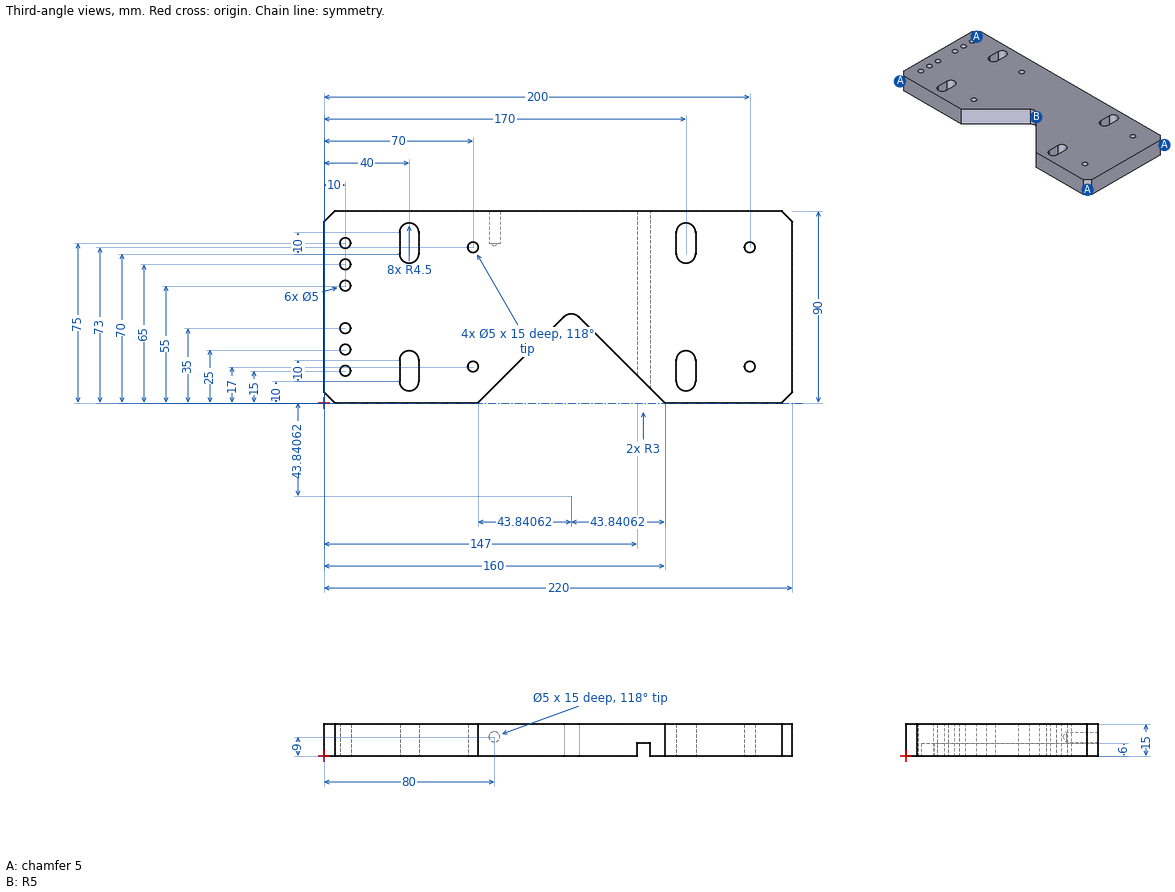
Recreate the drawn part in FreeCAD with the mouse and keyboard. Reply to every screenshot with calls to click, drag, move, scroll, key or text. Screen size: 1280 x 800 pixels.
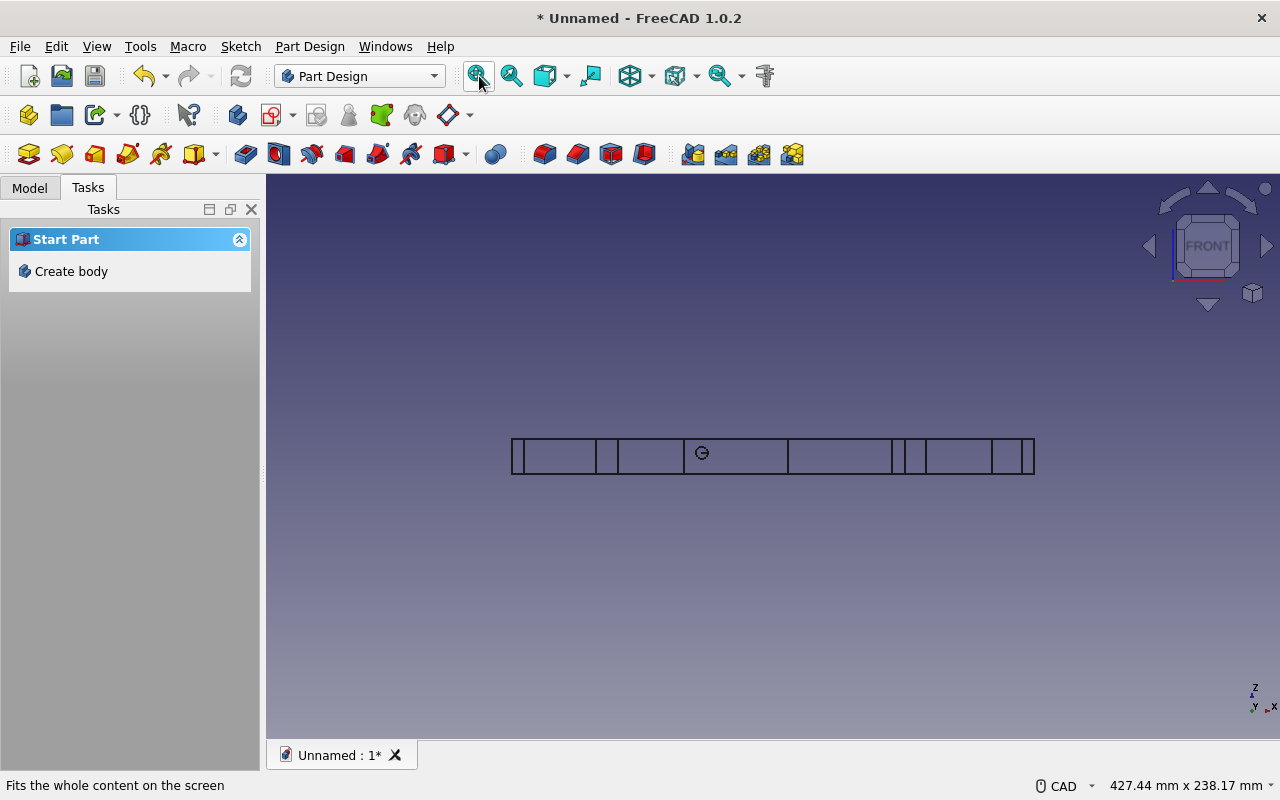
click(788, 455)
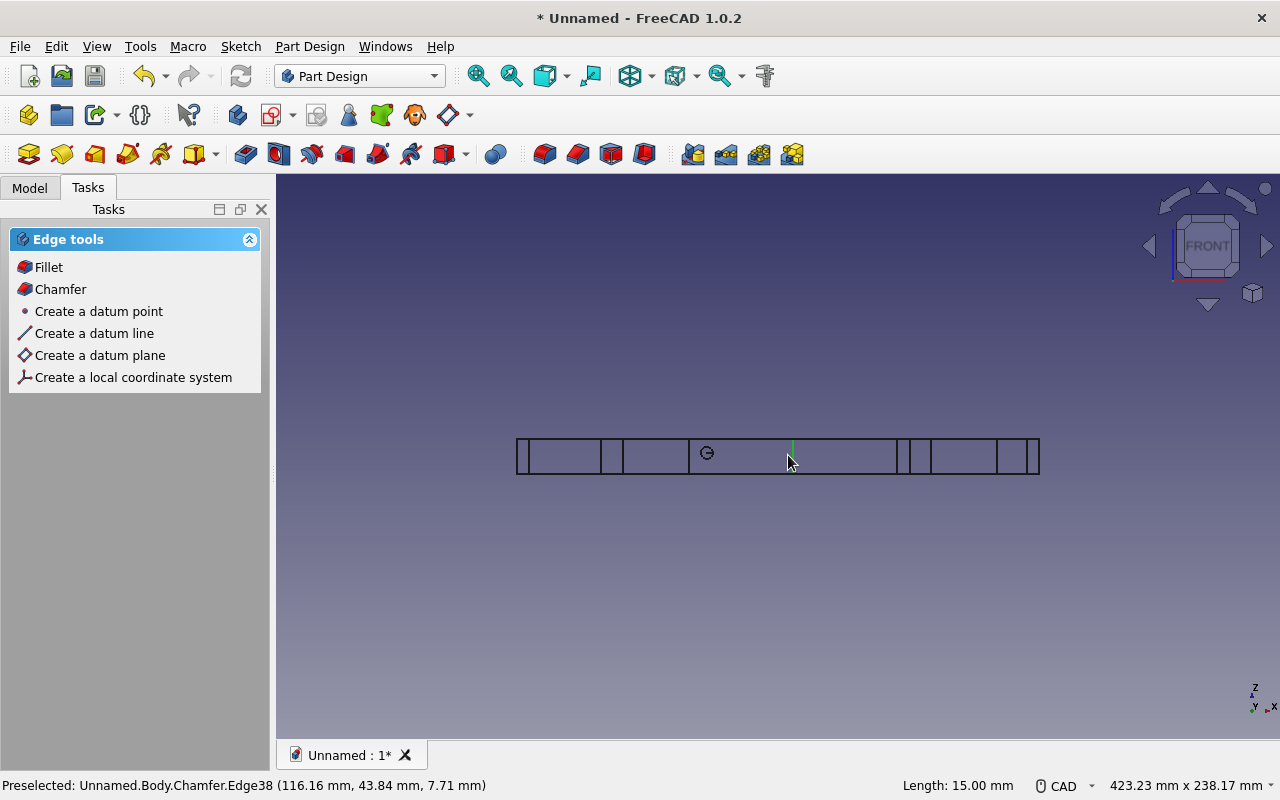
key(v)
key(1)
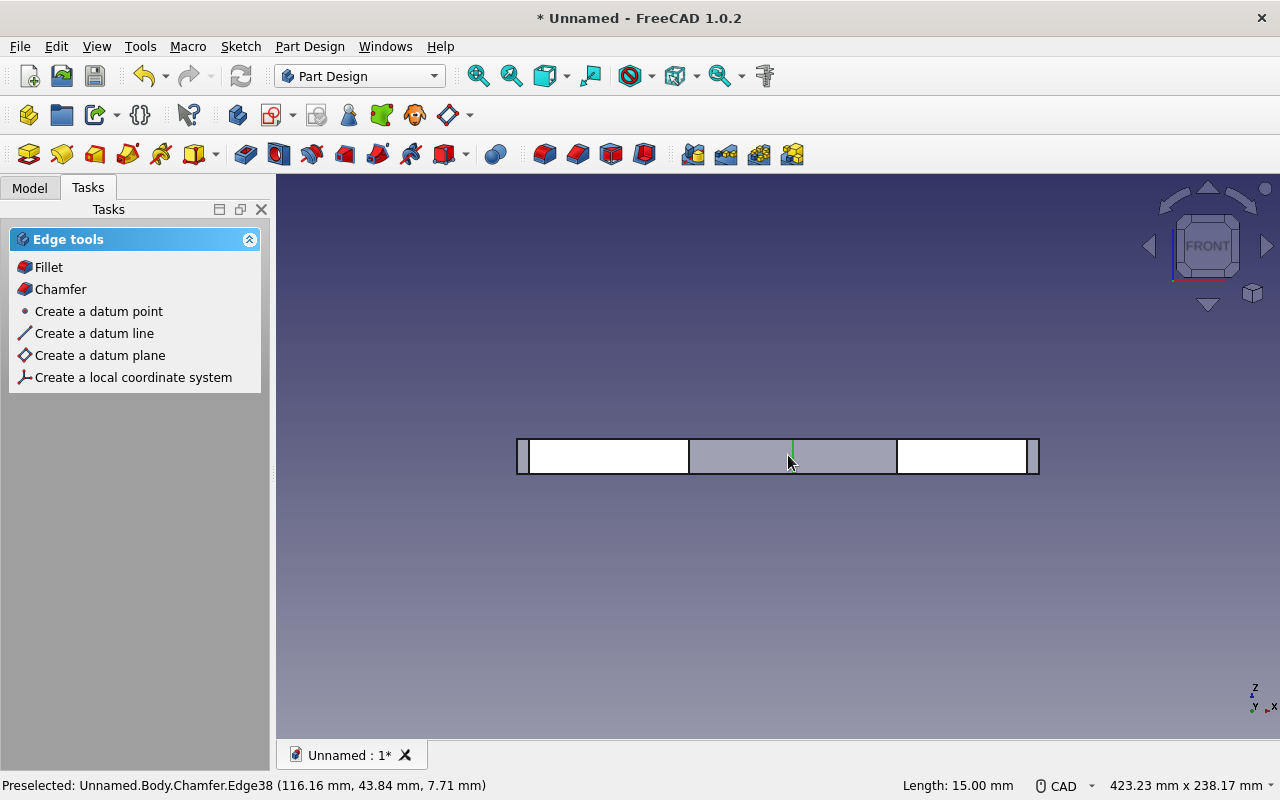
click(545, 154)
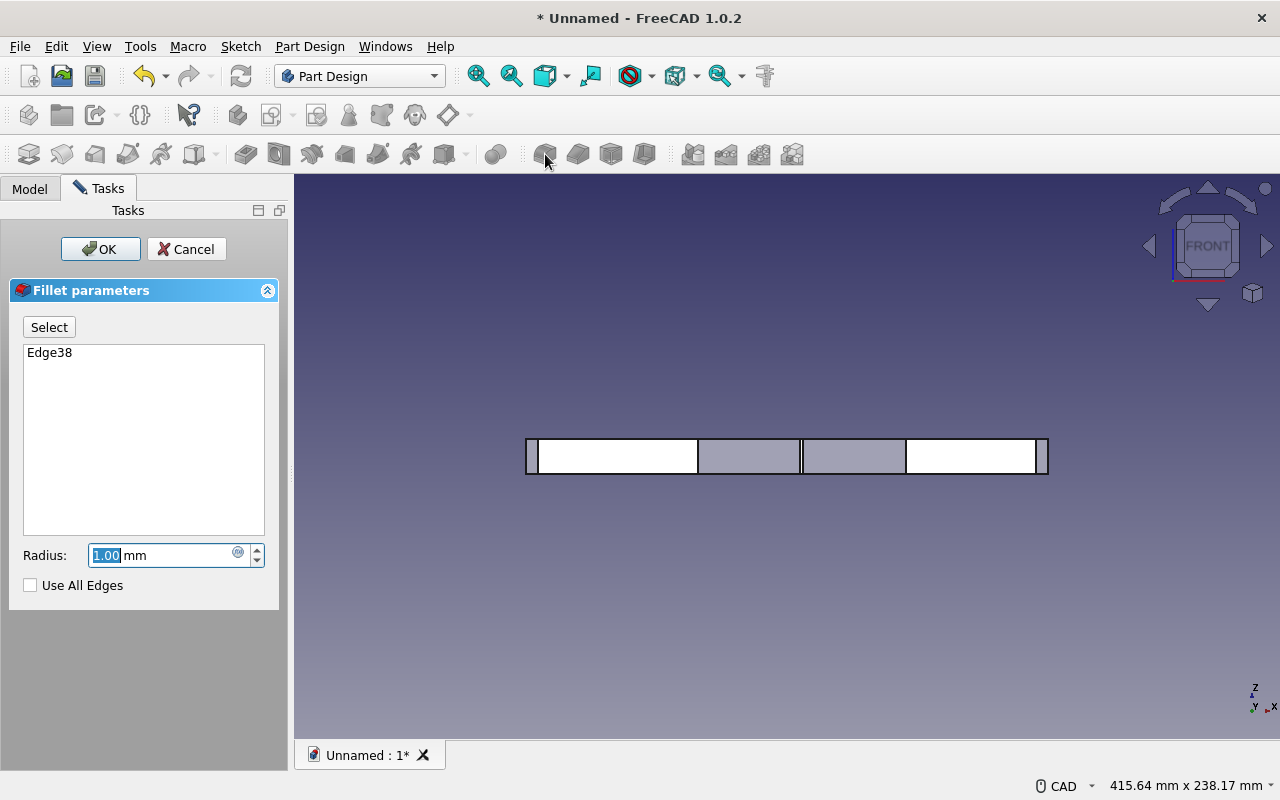
text(5)
key(Tab)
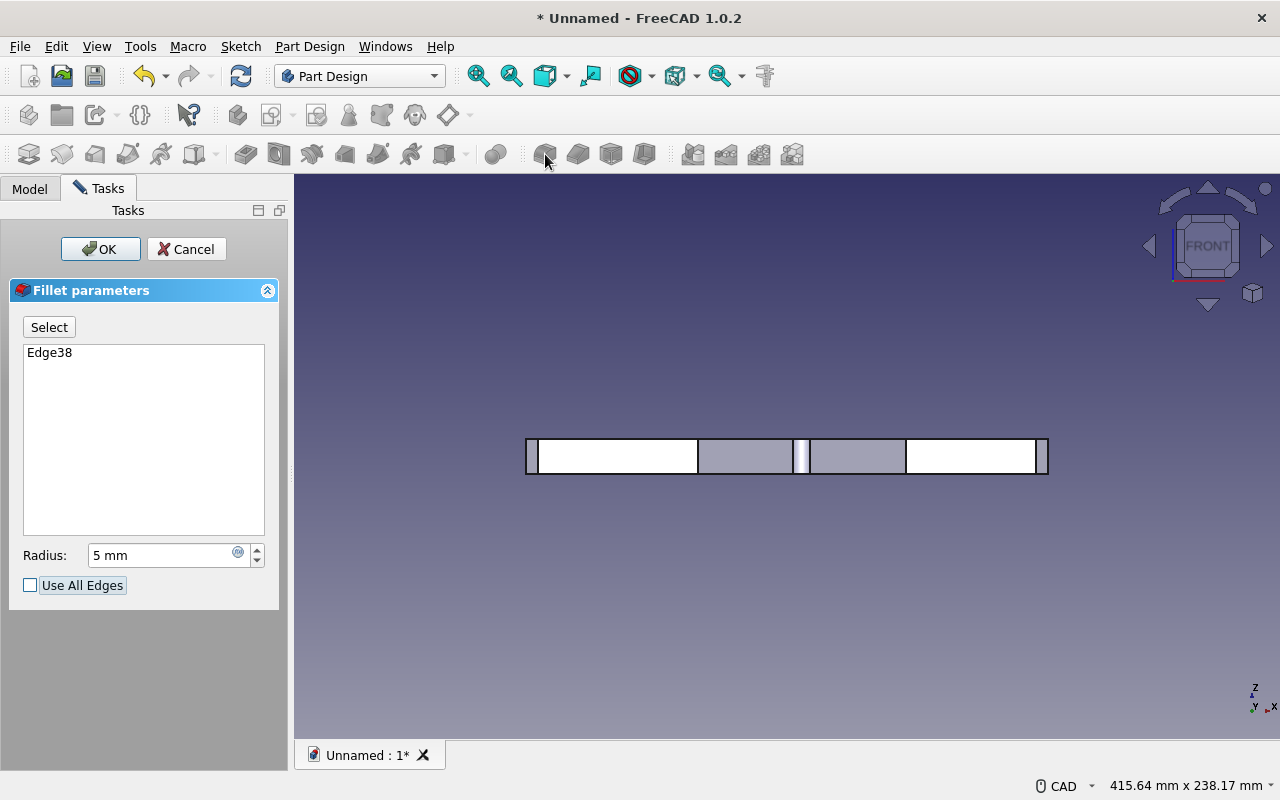
click(101, 249)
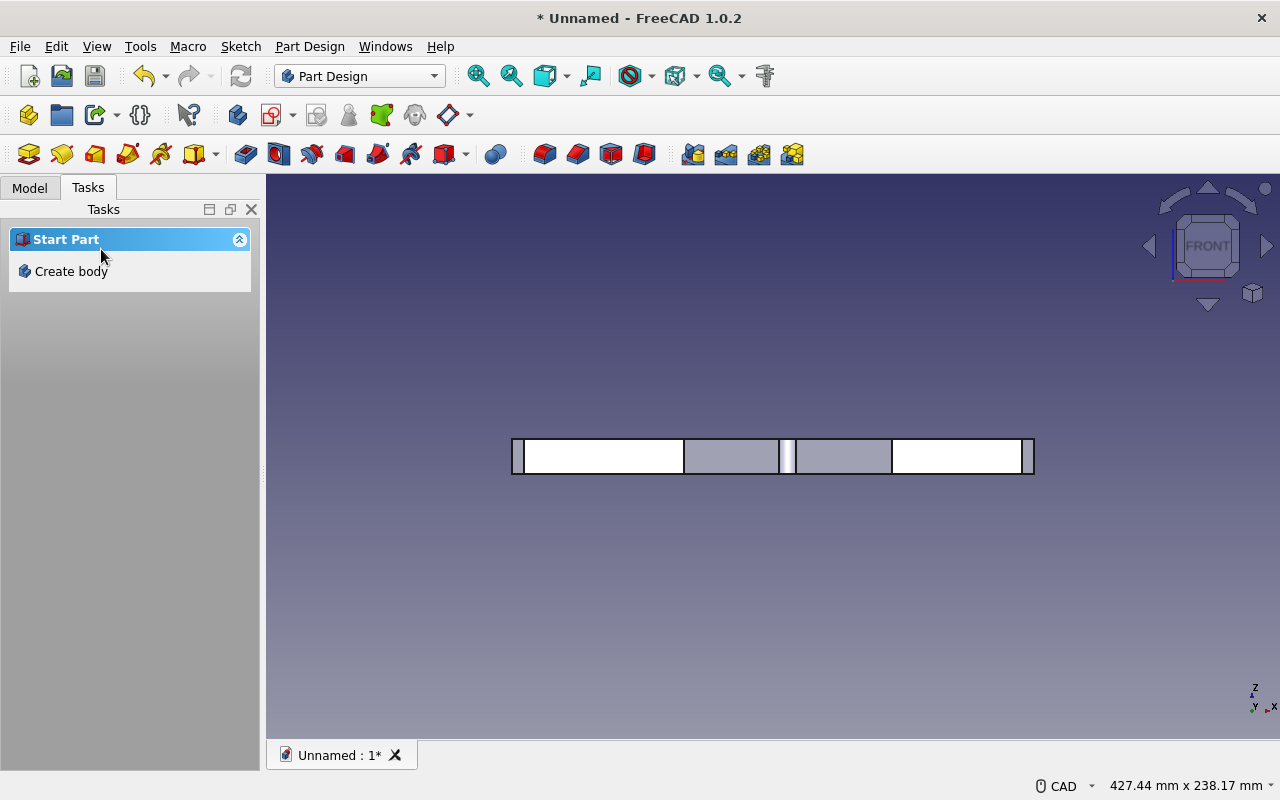
click(270, 116)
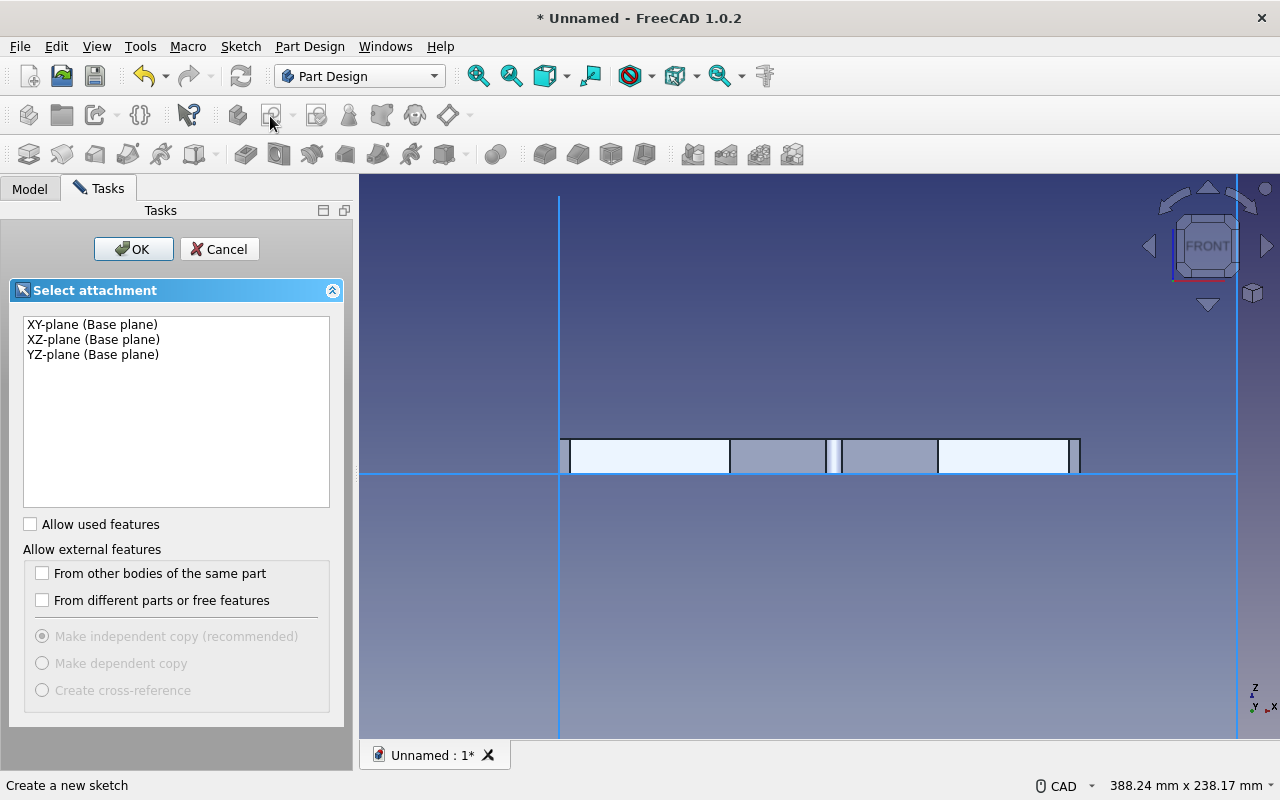
click(84, 324)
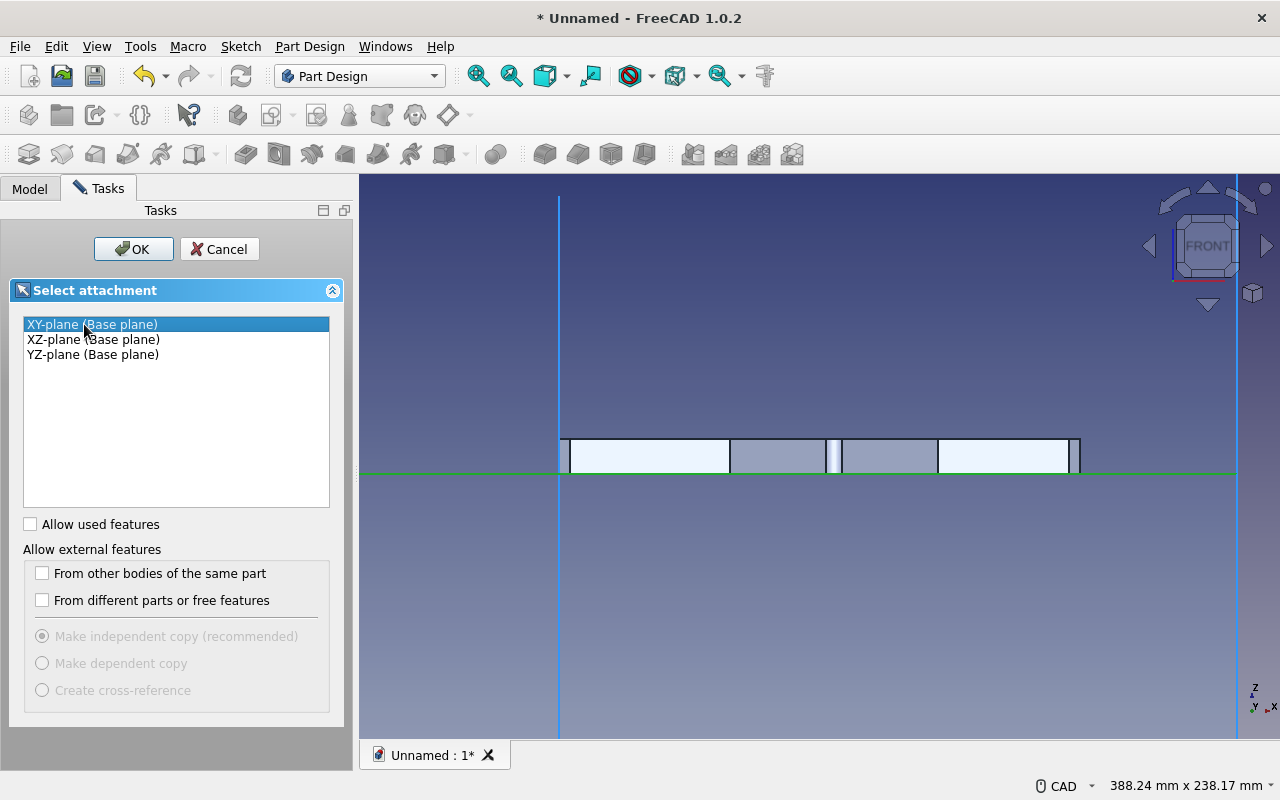
click(134, 249)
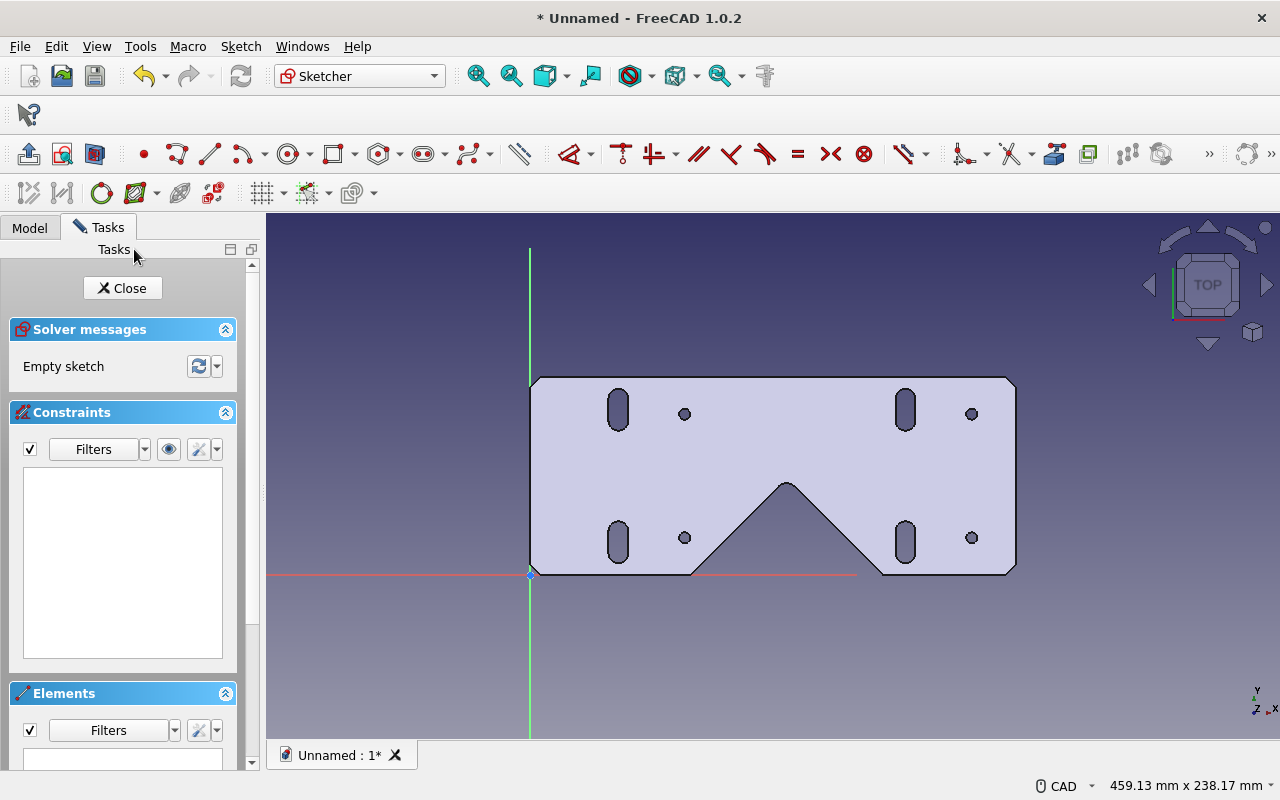
key(q)
key(s)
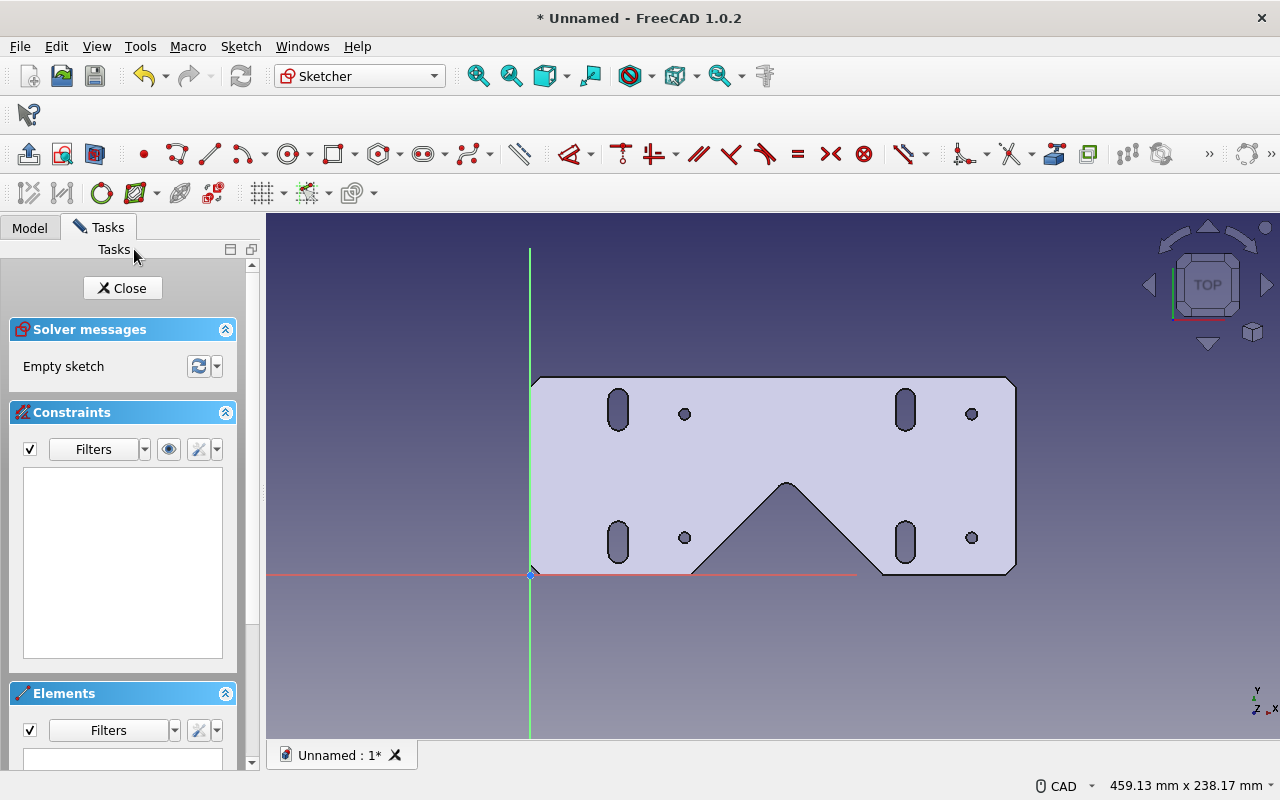
scroll(688, 476, up, 2)